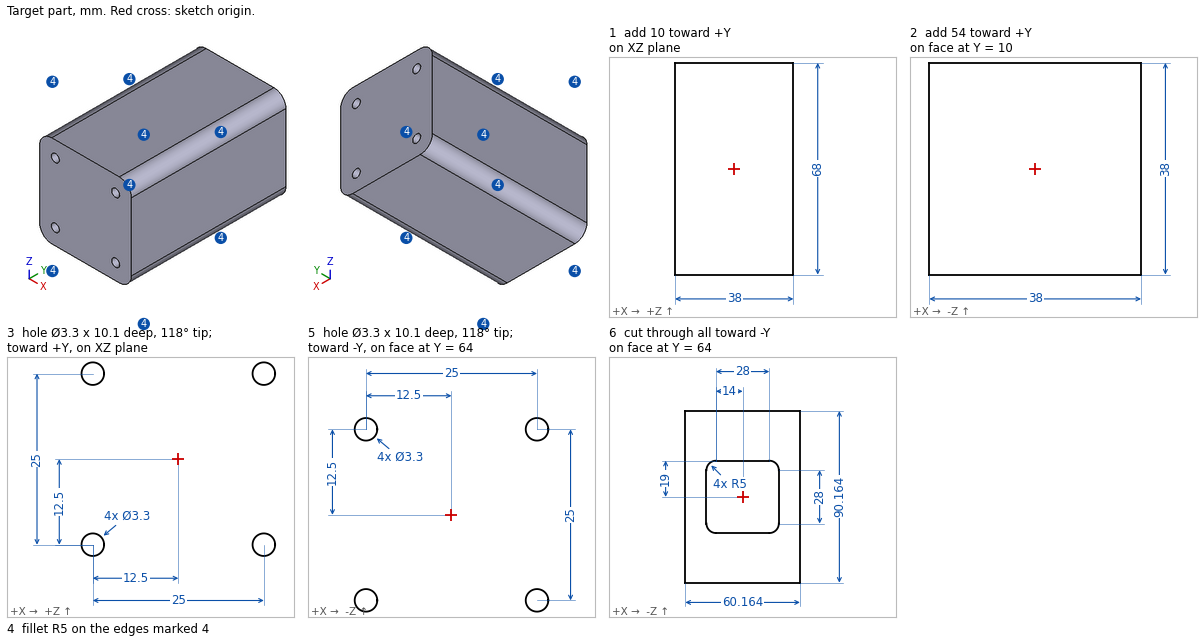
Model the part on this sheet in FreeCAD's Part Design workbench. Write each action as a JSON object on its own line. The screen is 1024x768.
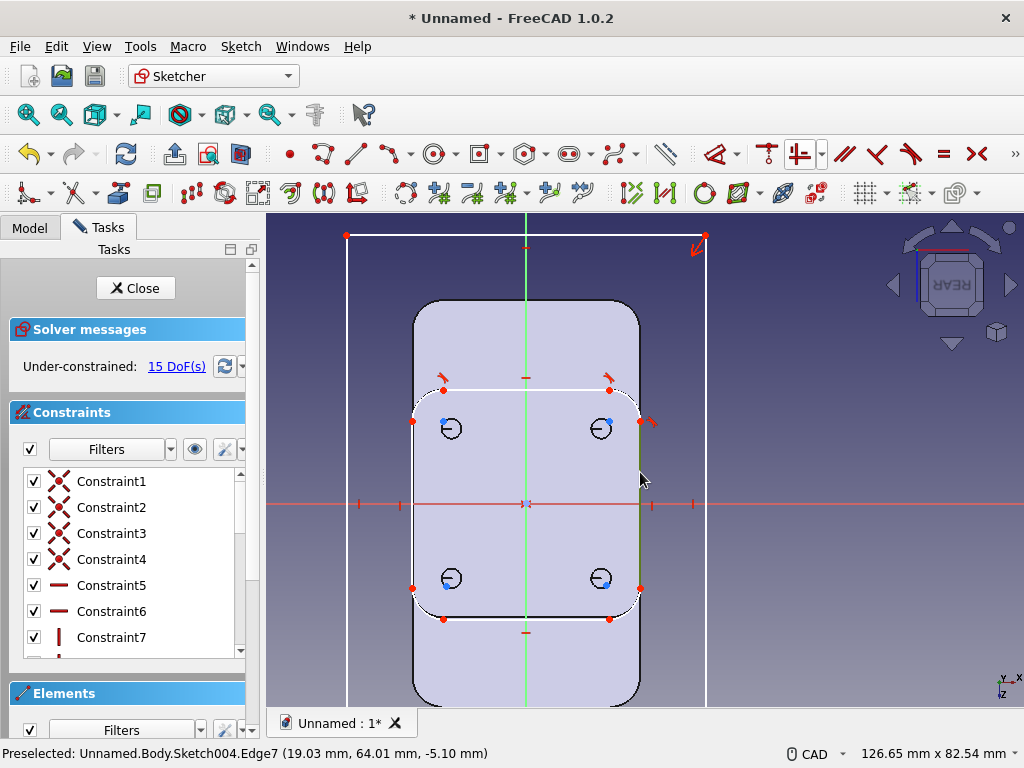
{"action": "left_click", "coordinate": [623, 616]}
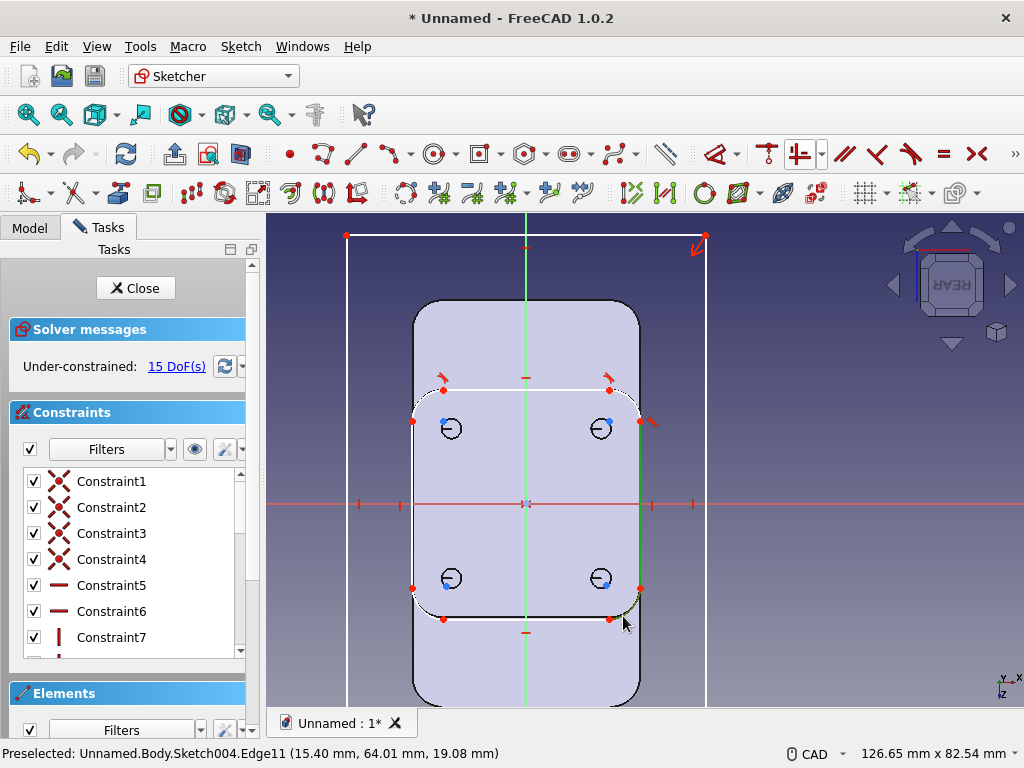
{"action": "key", "text": "t"}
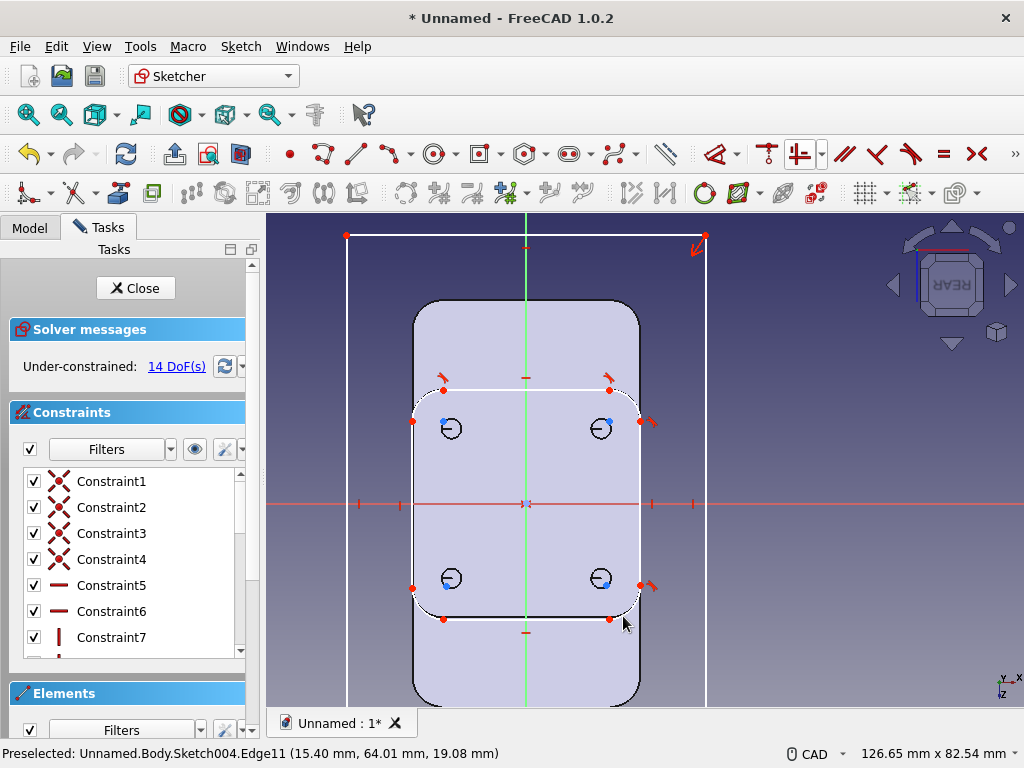
{"action": "left_click", "coordinate": [560, 620]}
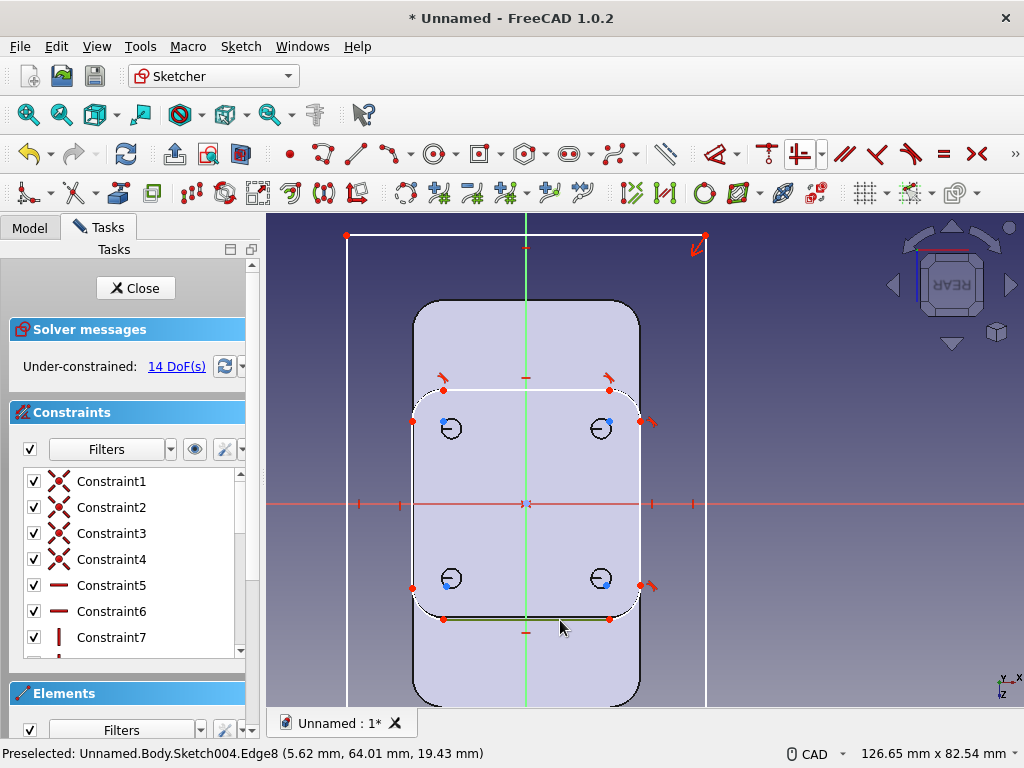
{"action": "left_click", "coordinate": [624, 615]}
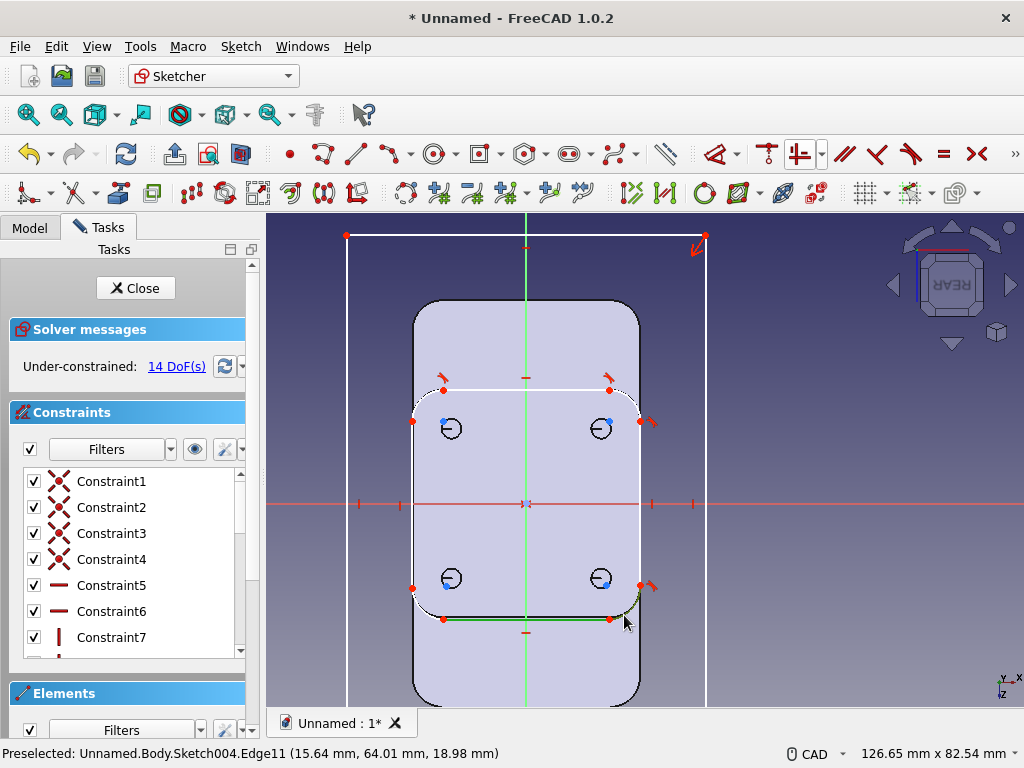
{"action": "key", "text": "t"}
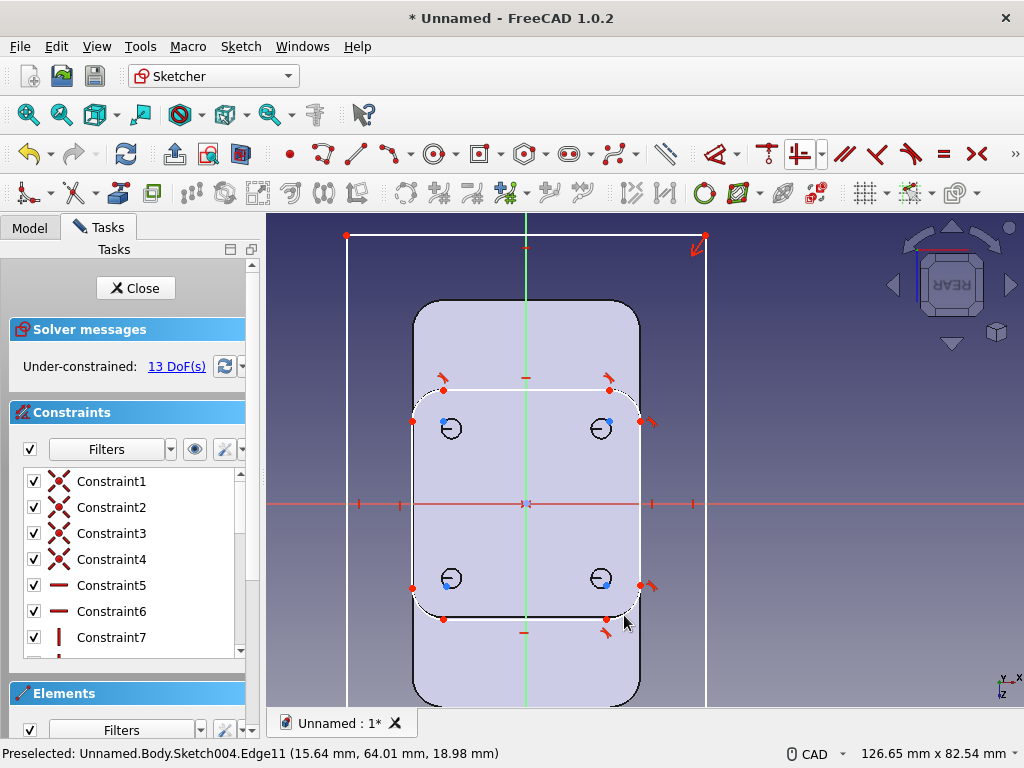
{"action": "left_click", "coordinate": [557, 620]}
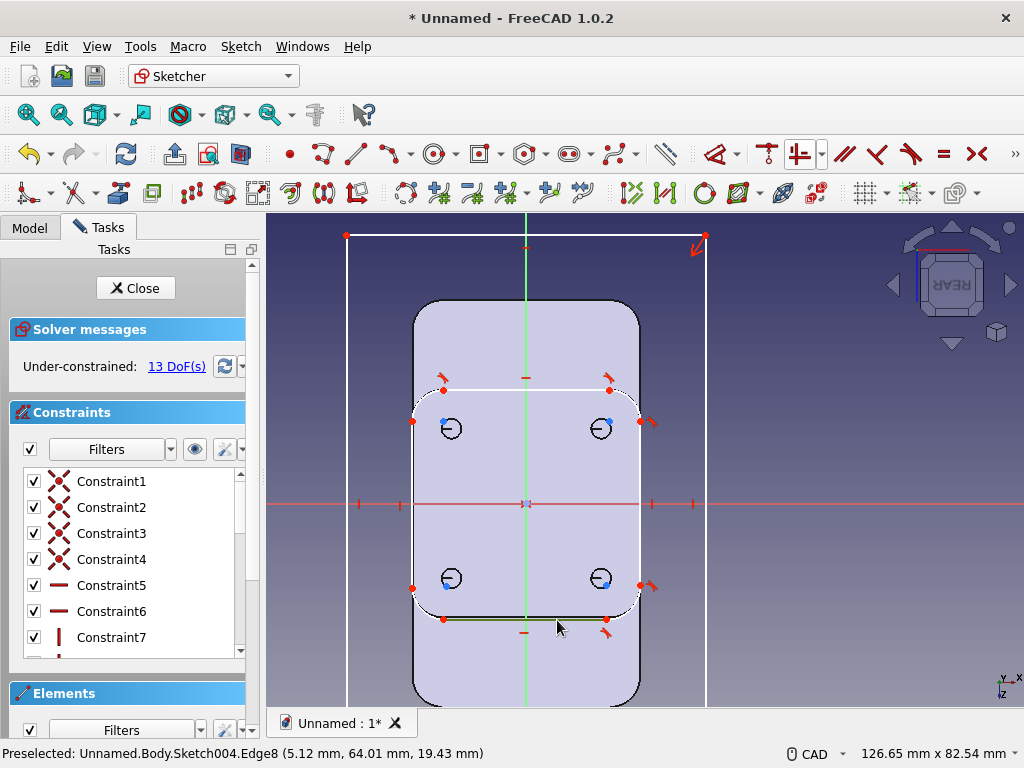
{"action": "left_click", "coordinate": [417, 602]}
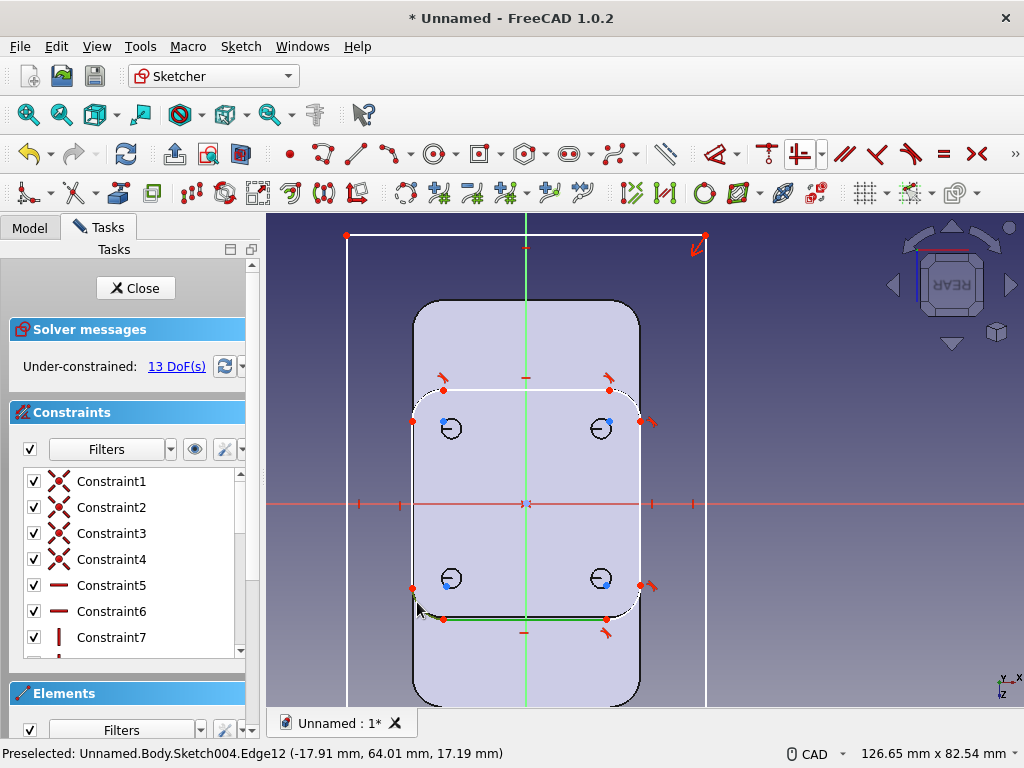
{"action": "left_click", "coordinate": [911, 154]}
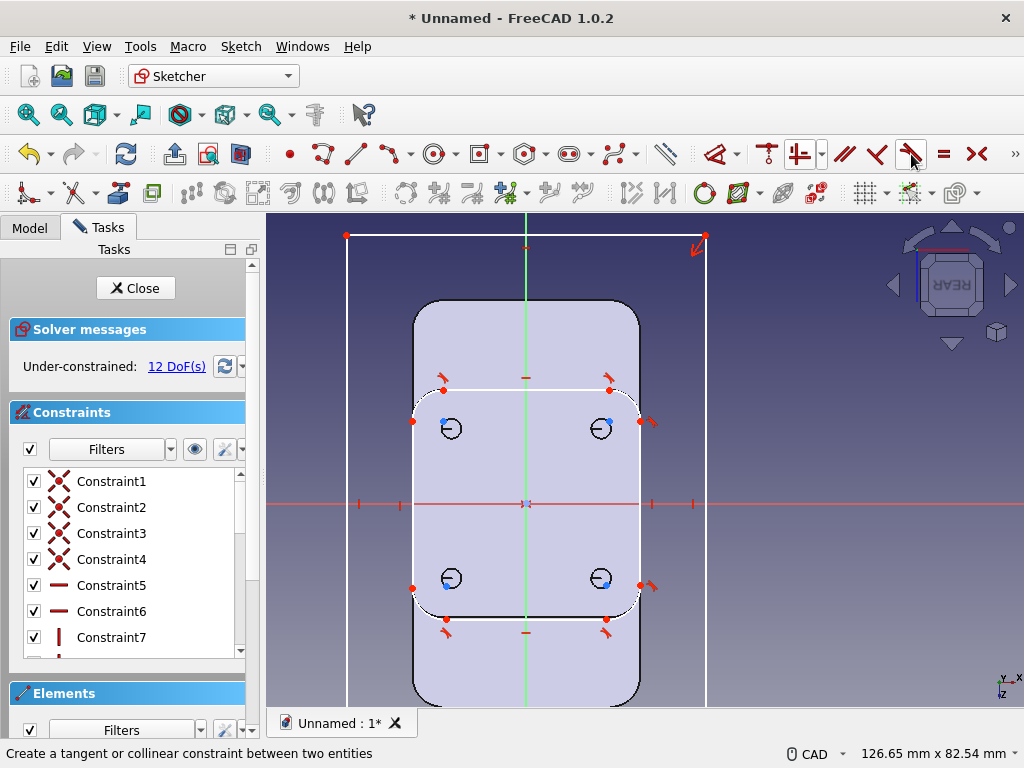
{"action": "left_click", "coordinate": [413, 539]}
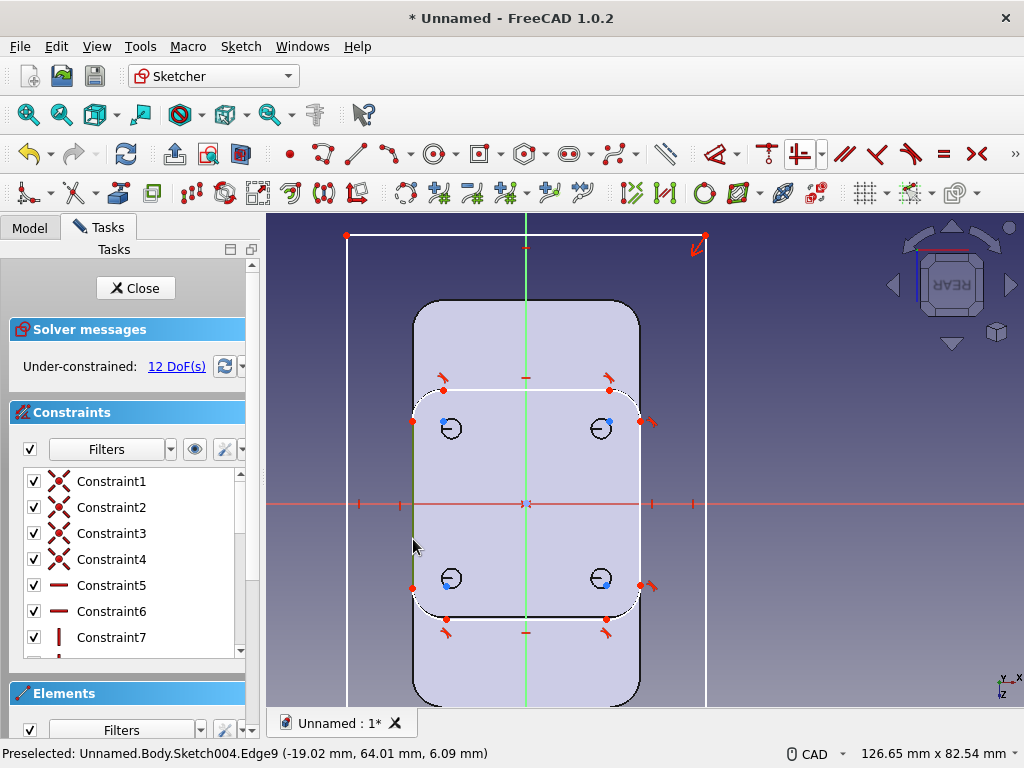
{"action": "left_click", "coordinate": [417, 603]}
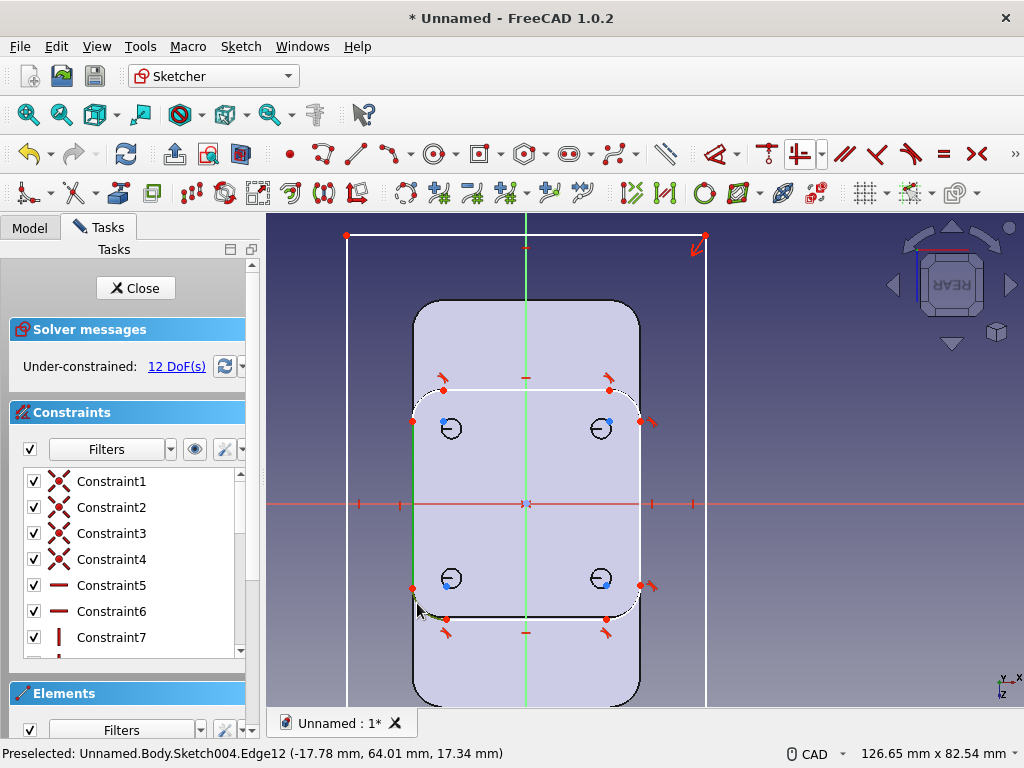
{"action": "left_click", "coordinate": [911, 154]}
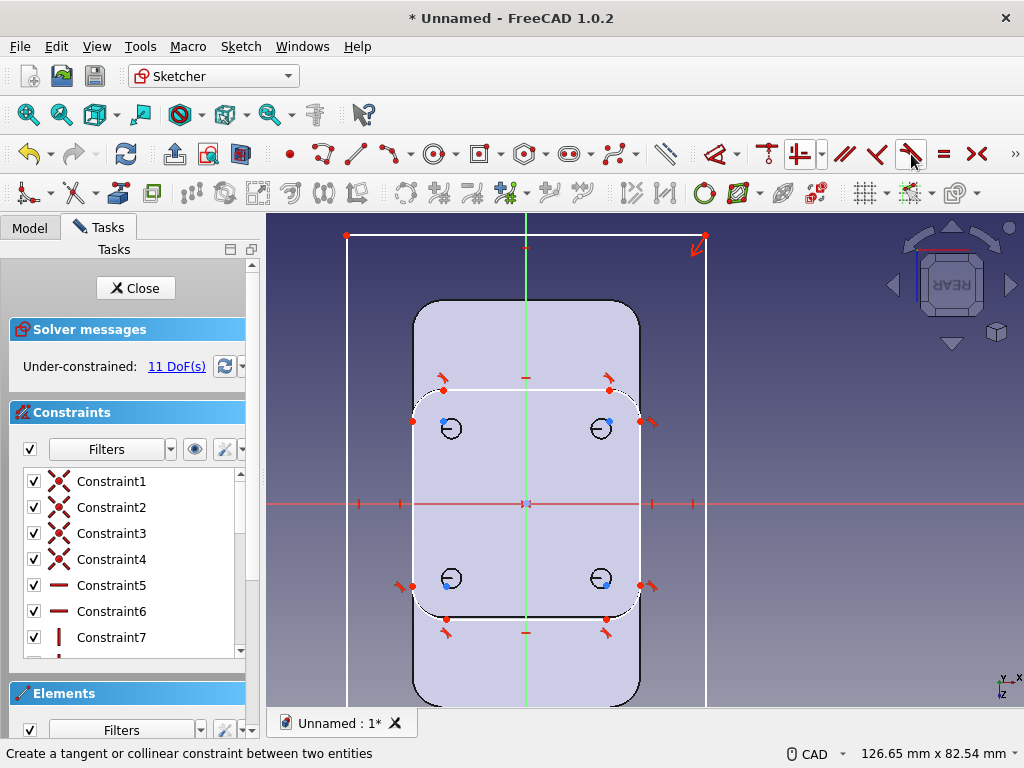
{"action": "left_click", "coordinate": [413, 537]}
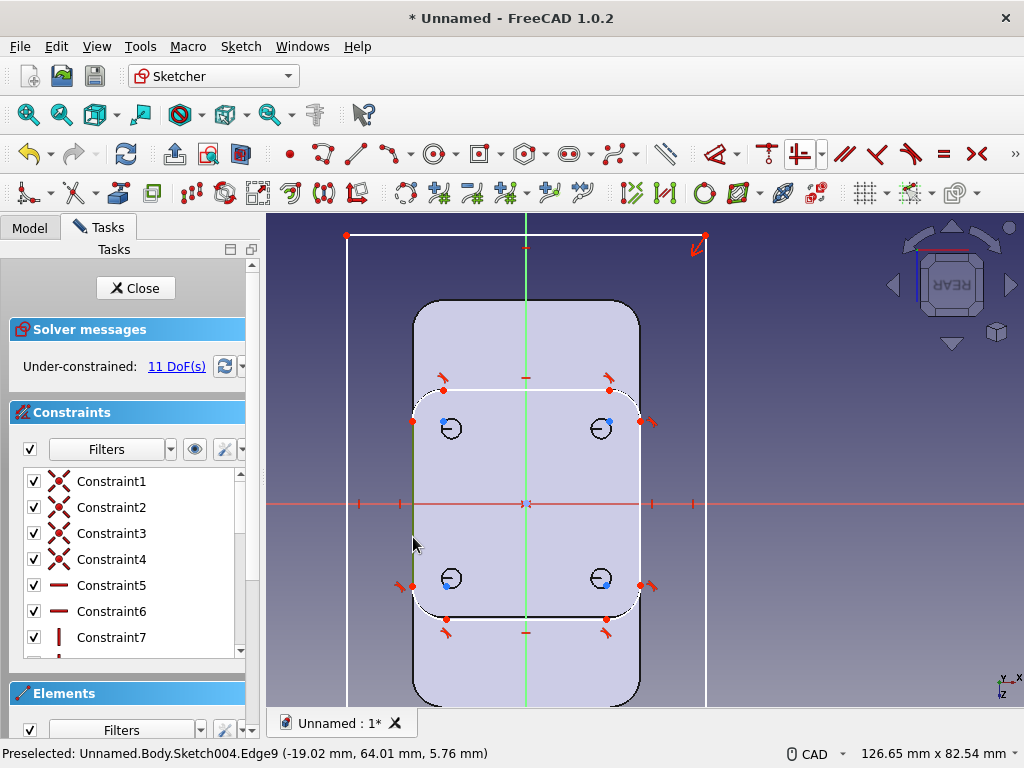
{"action": "left_click", "coordinate": [429, 394]}